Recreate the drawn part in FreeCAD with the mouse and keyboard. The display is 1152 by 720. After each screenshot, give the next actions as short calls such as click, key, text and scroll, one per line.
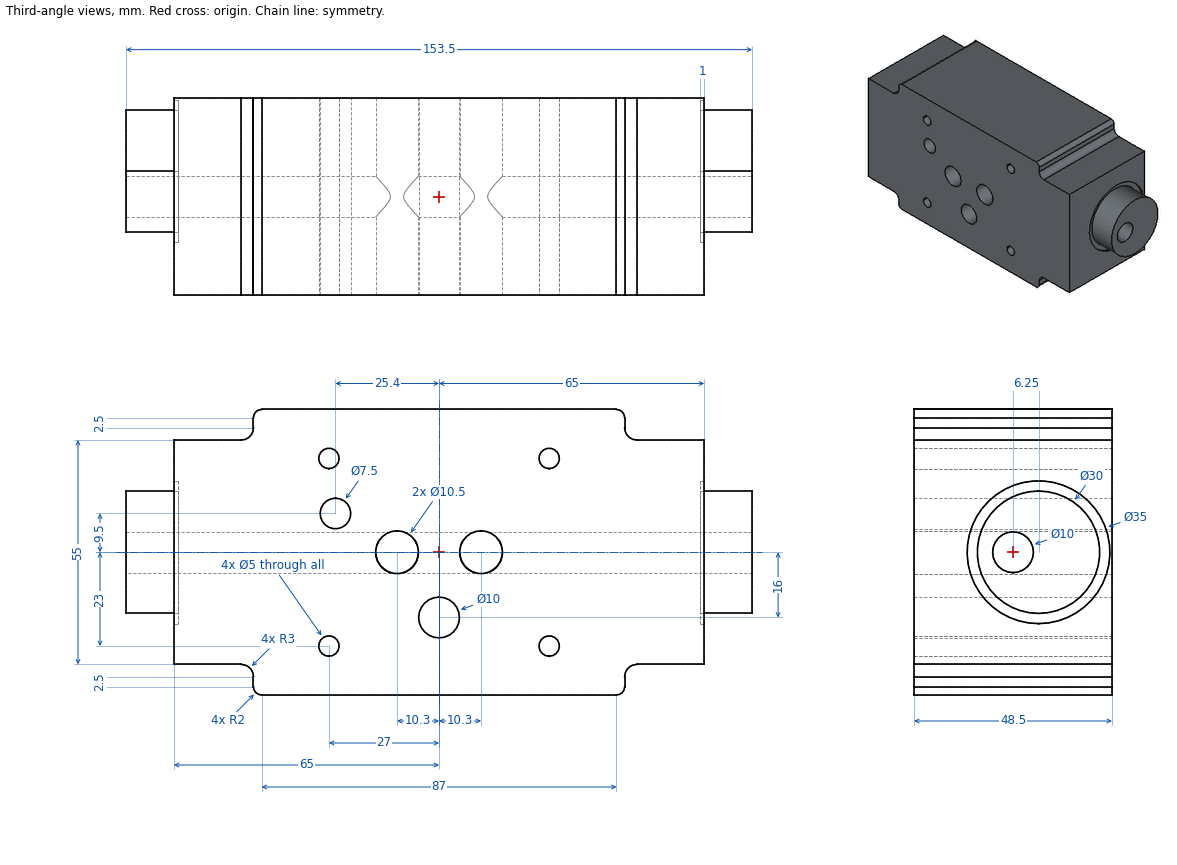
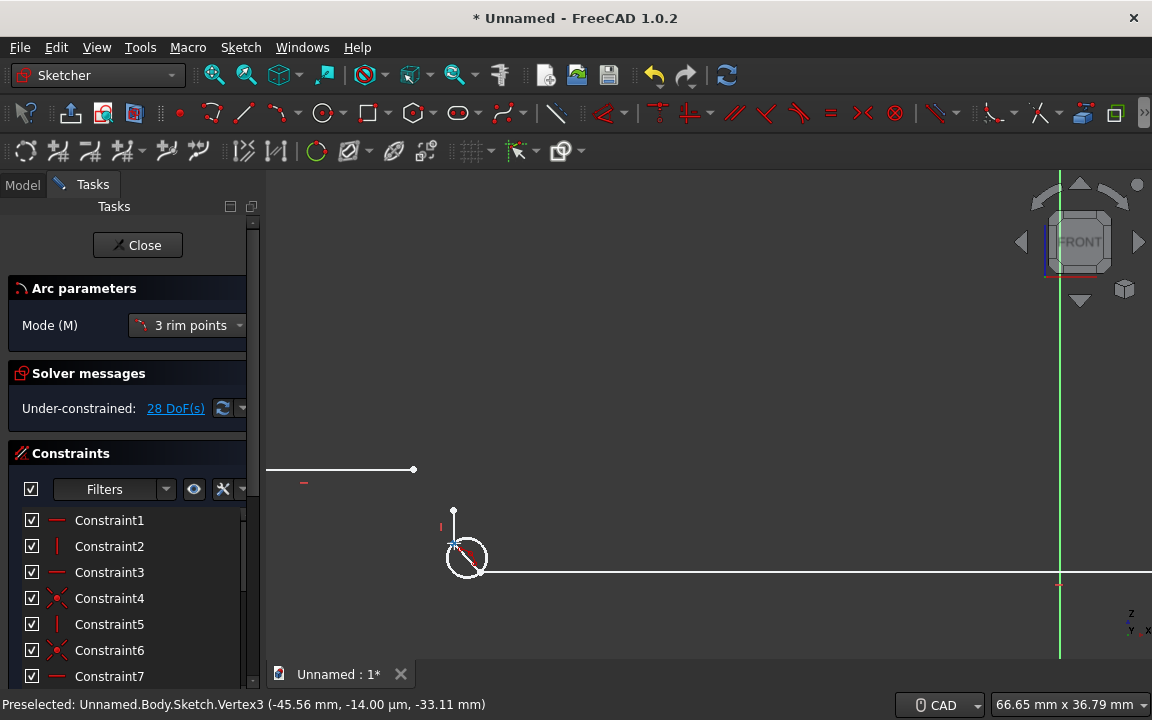
scroll(463, 561, up, 4)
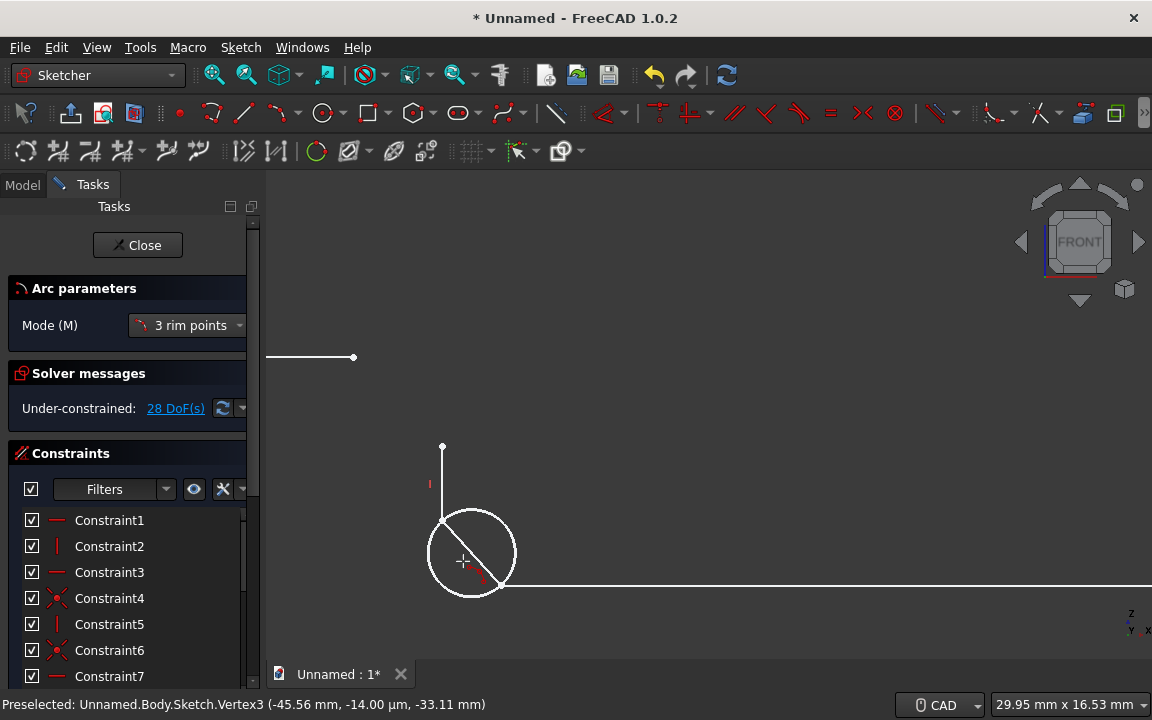
click(462, 559)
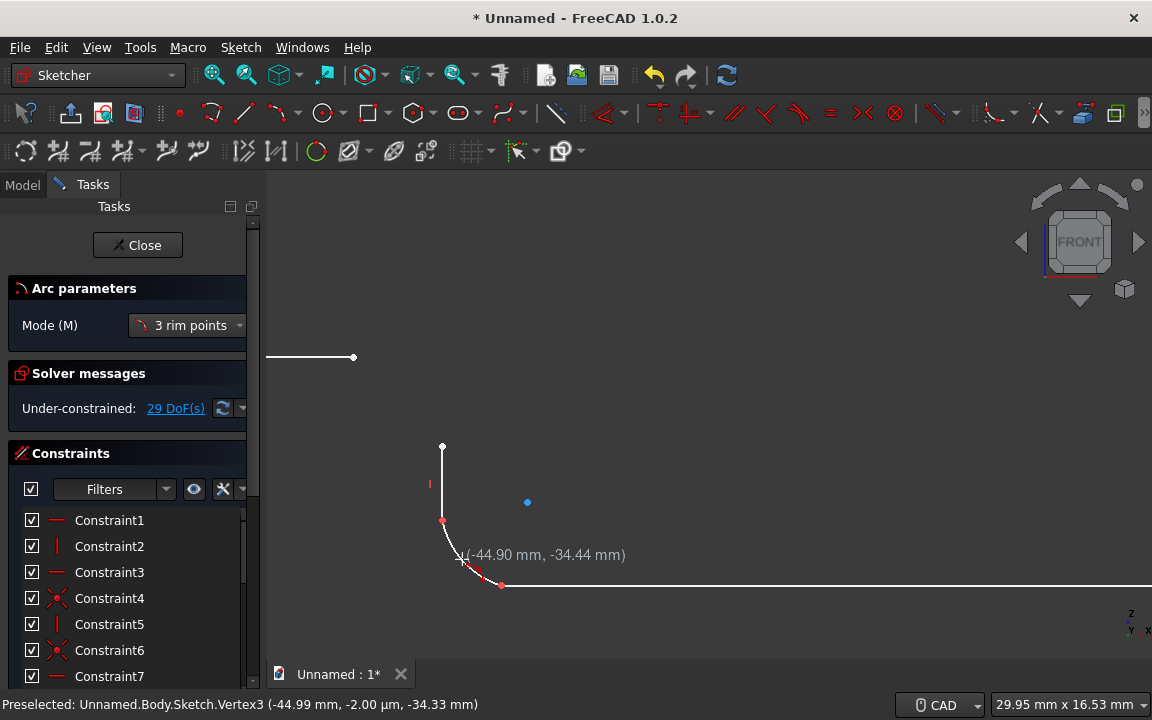
click(442, 447)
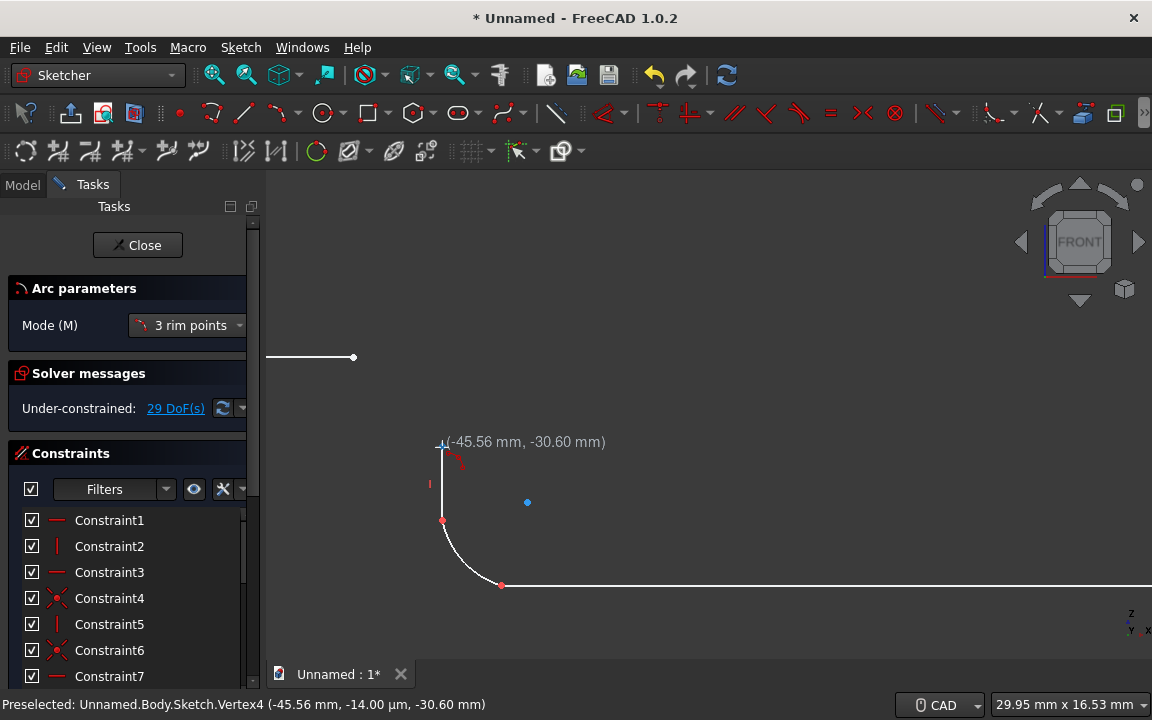
scroll(461, 551, down, 10)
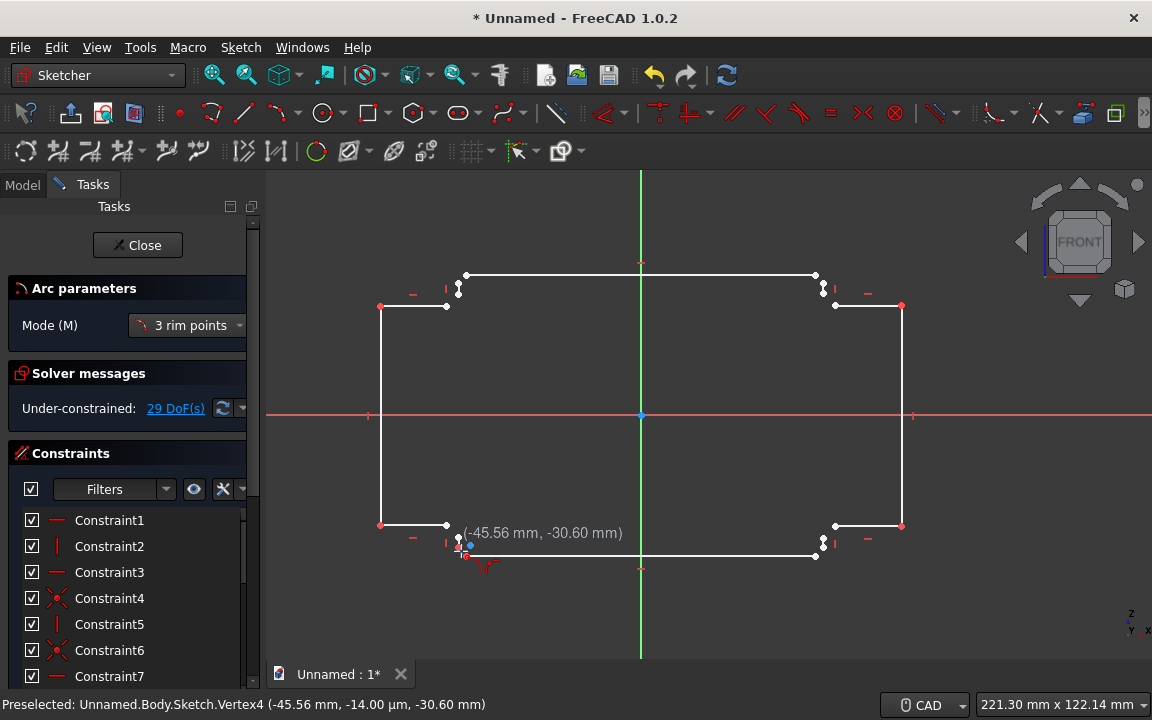
click(447, 525)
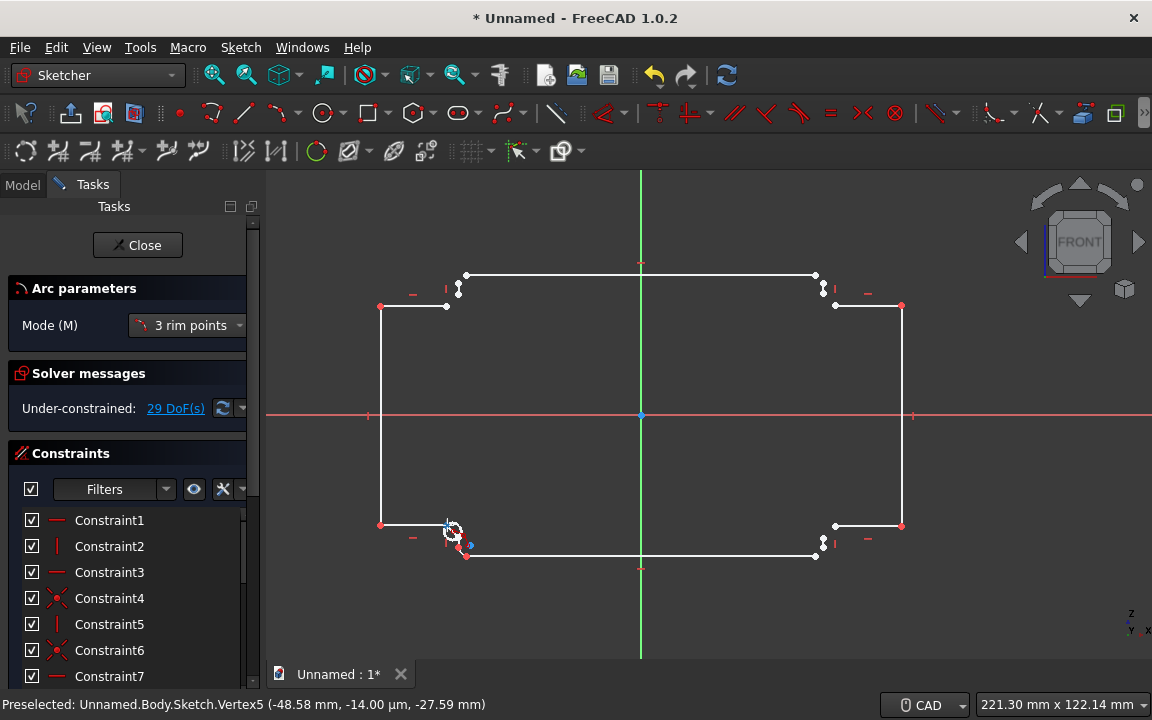
scroll(455, 529, up, 8)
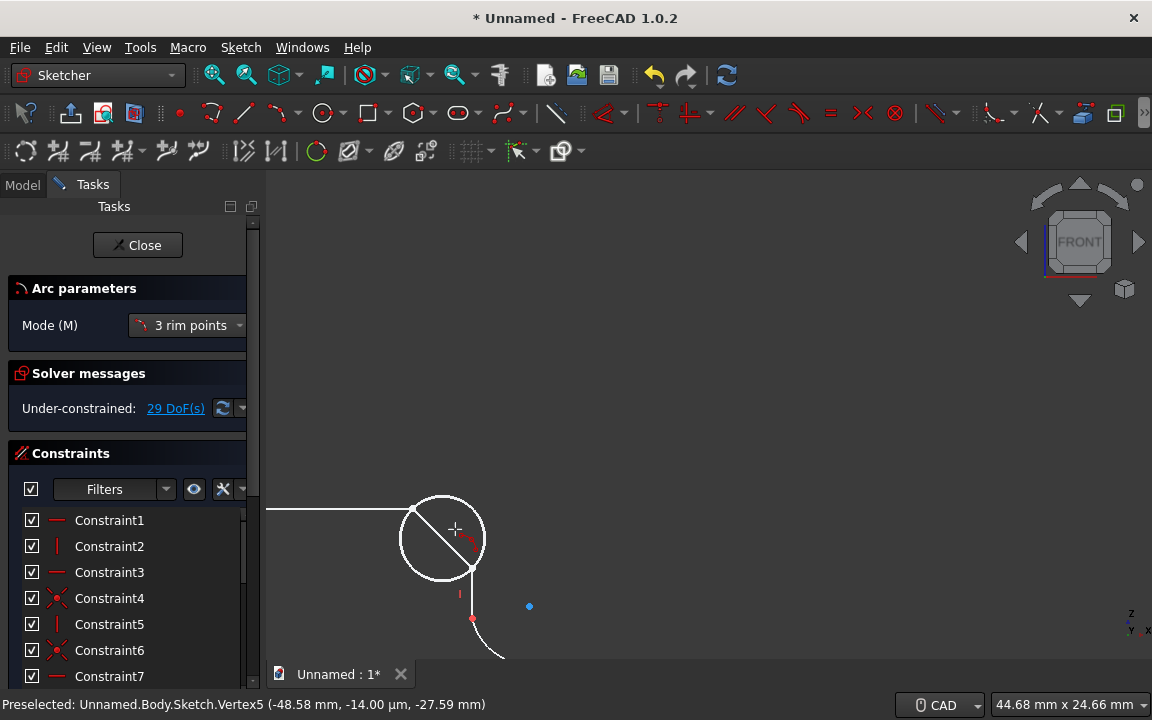
click(456, 524)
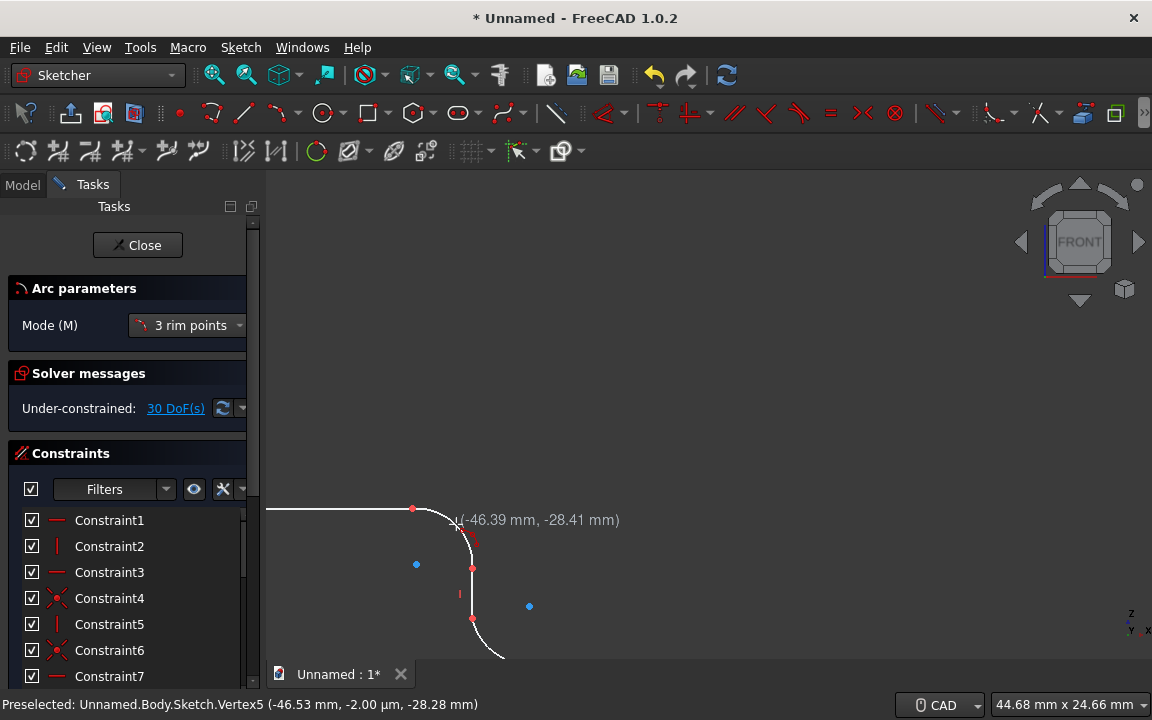
scroll(454, 529, down, 8)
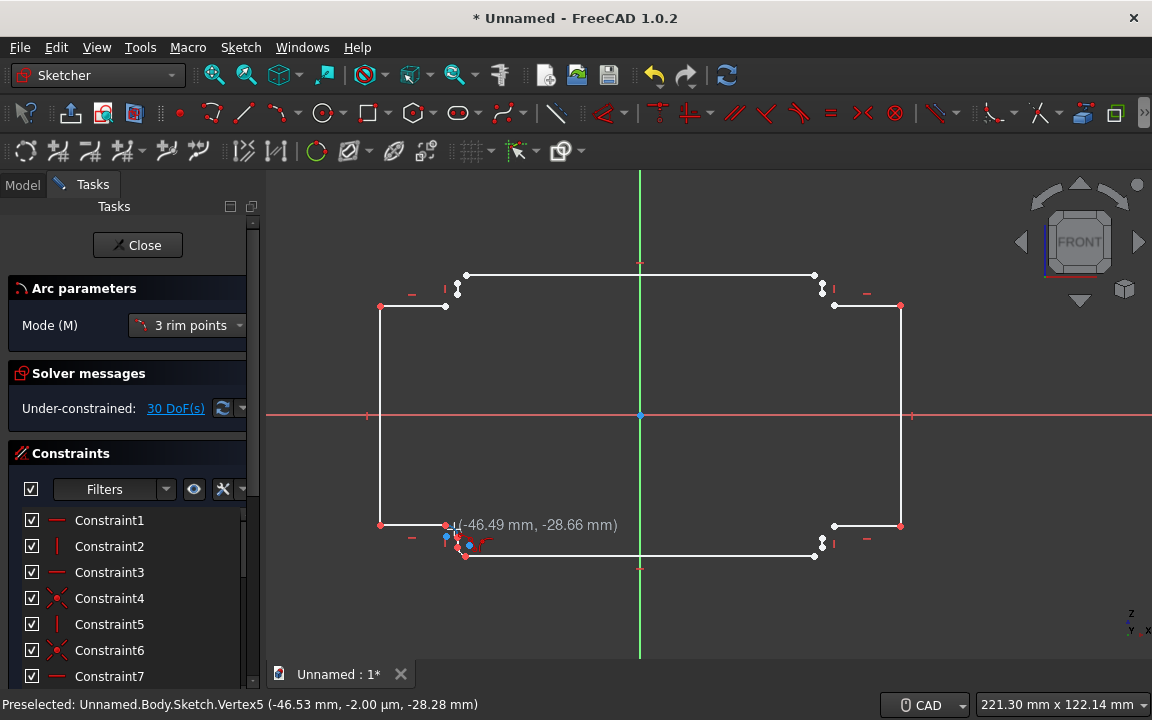
click(446, 306)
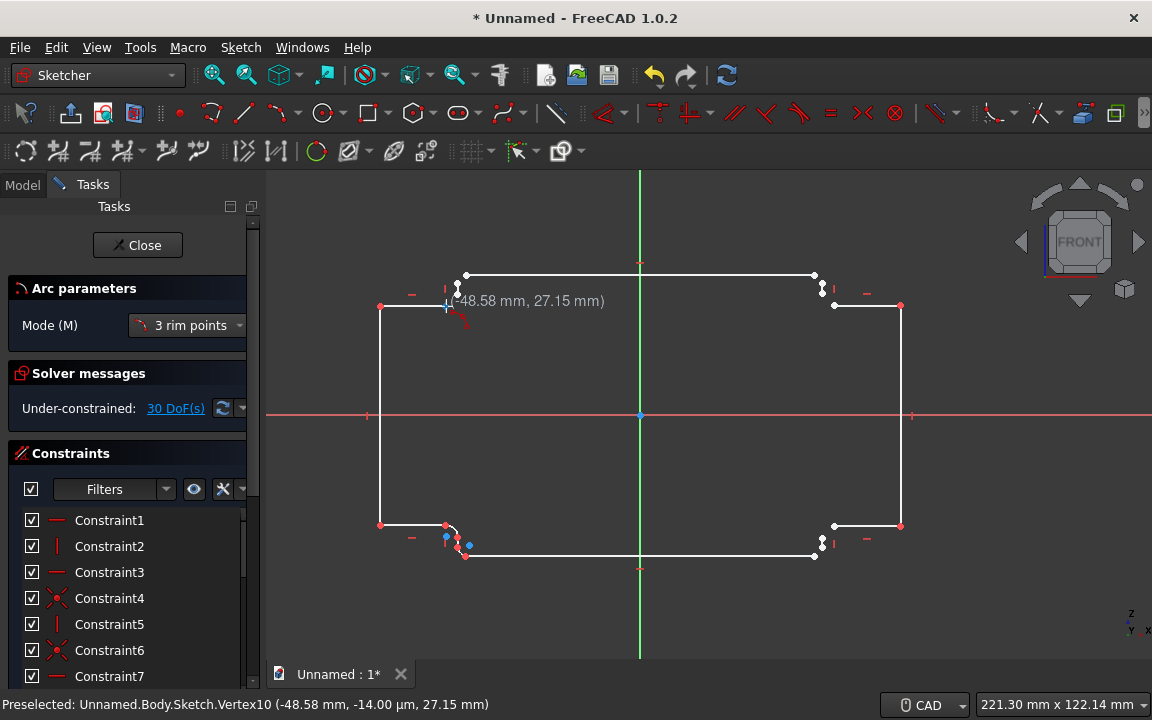
scroll(458, 293, up, 6)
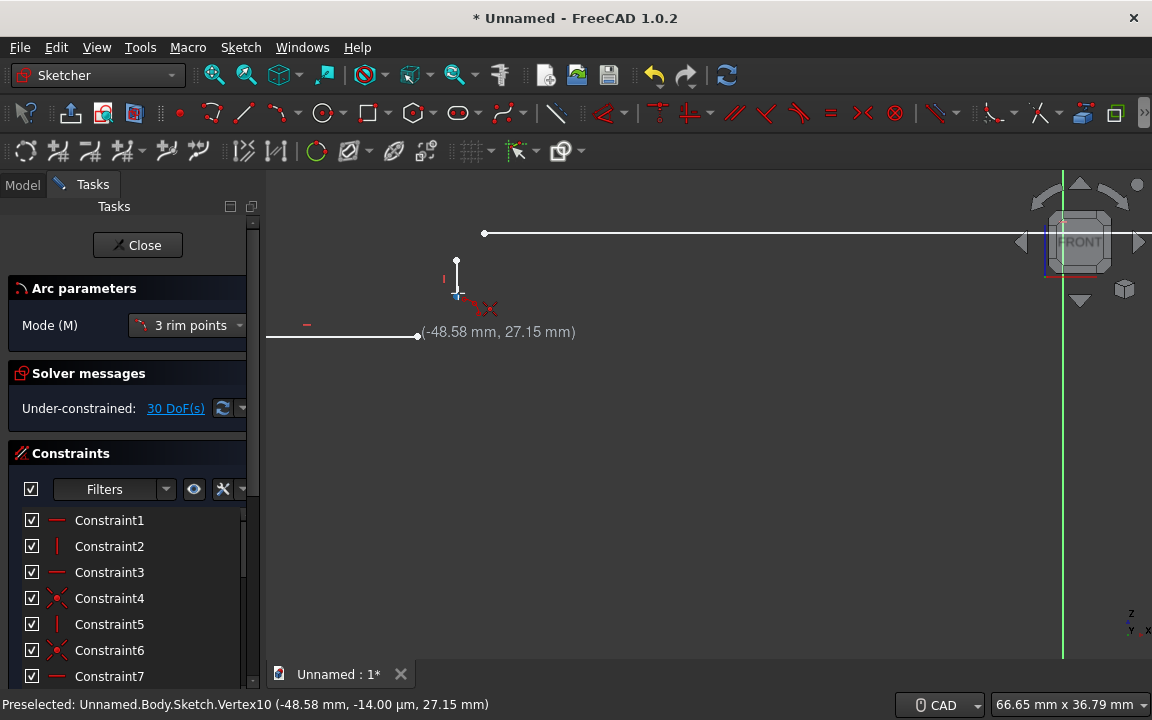
click(457, 297)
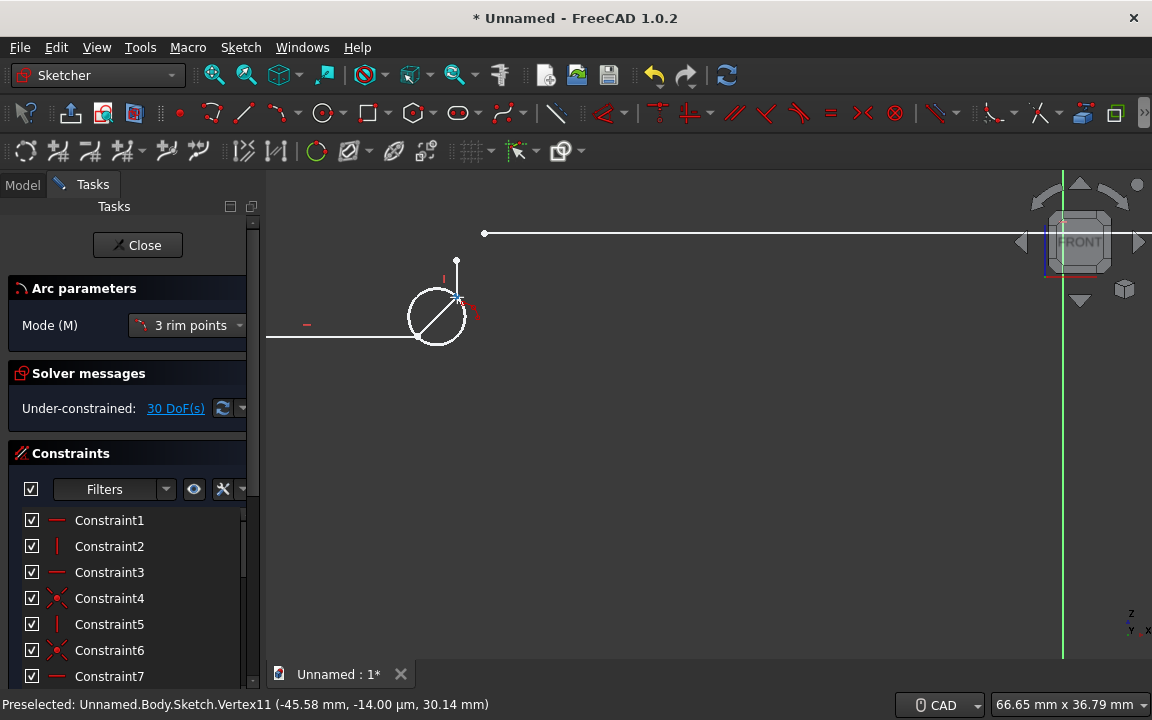
scroll(446, 320, up, 2)